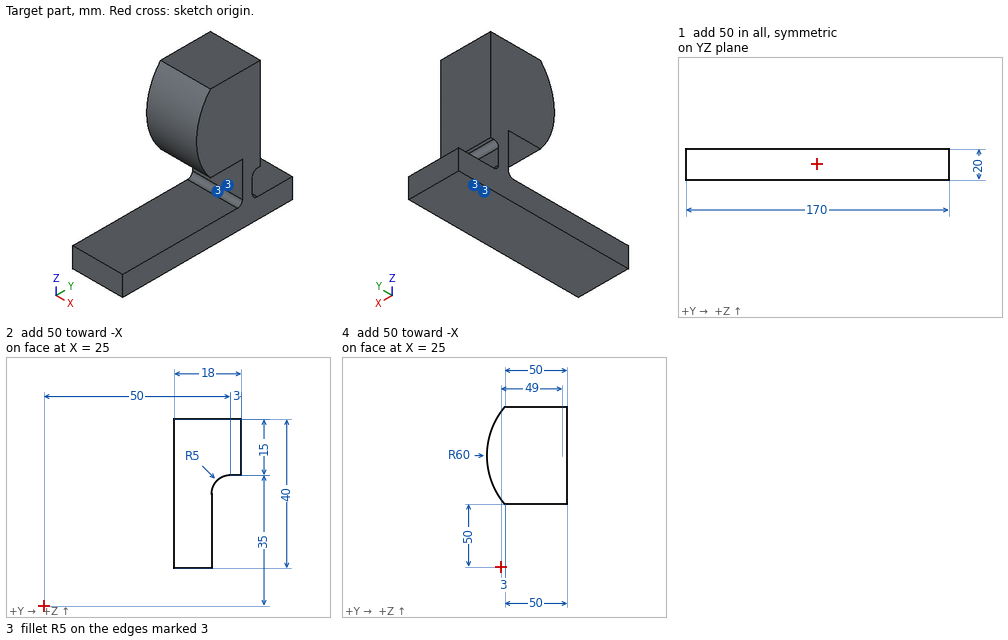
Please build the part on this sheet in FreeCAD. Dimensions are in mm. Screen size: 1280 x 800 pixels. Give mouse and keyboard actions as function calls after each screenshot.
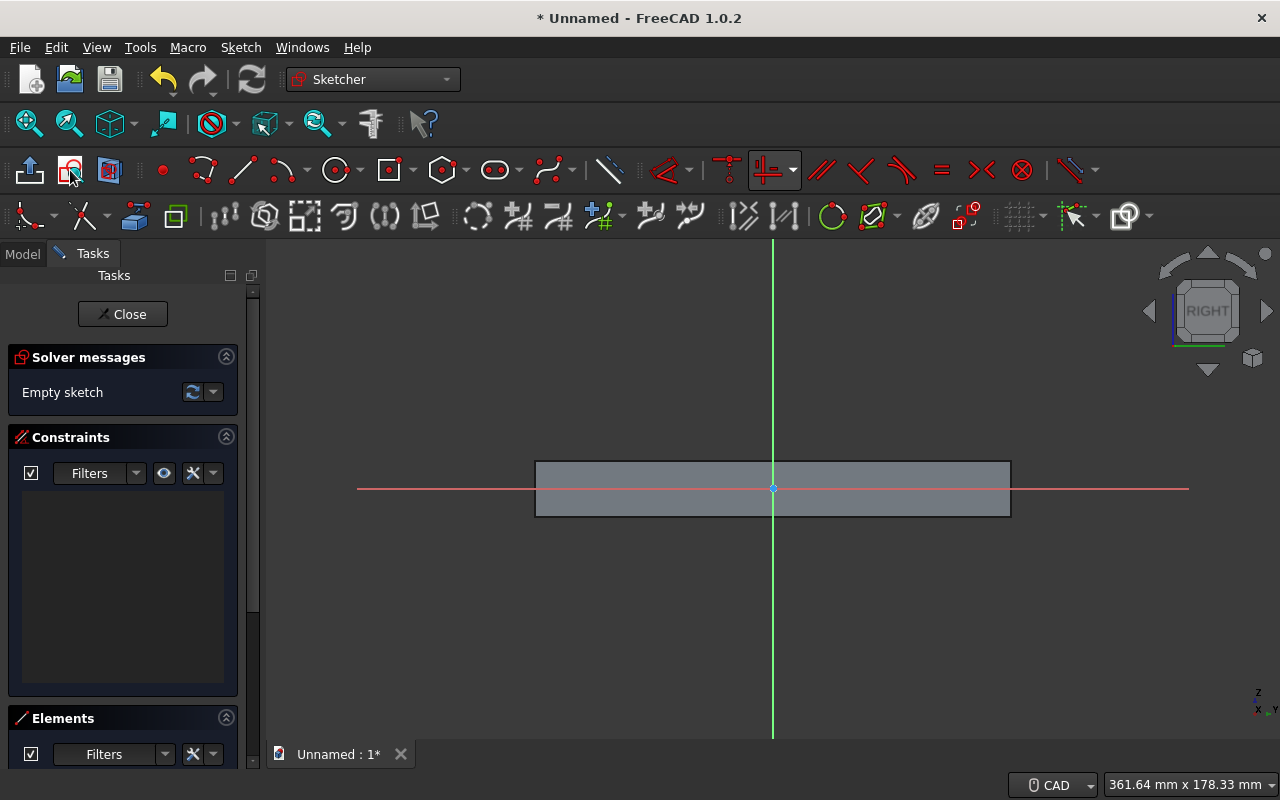
scroll(964, 362, up, 4)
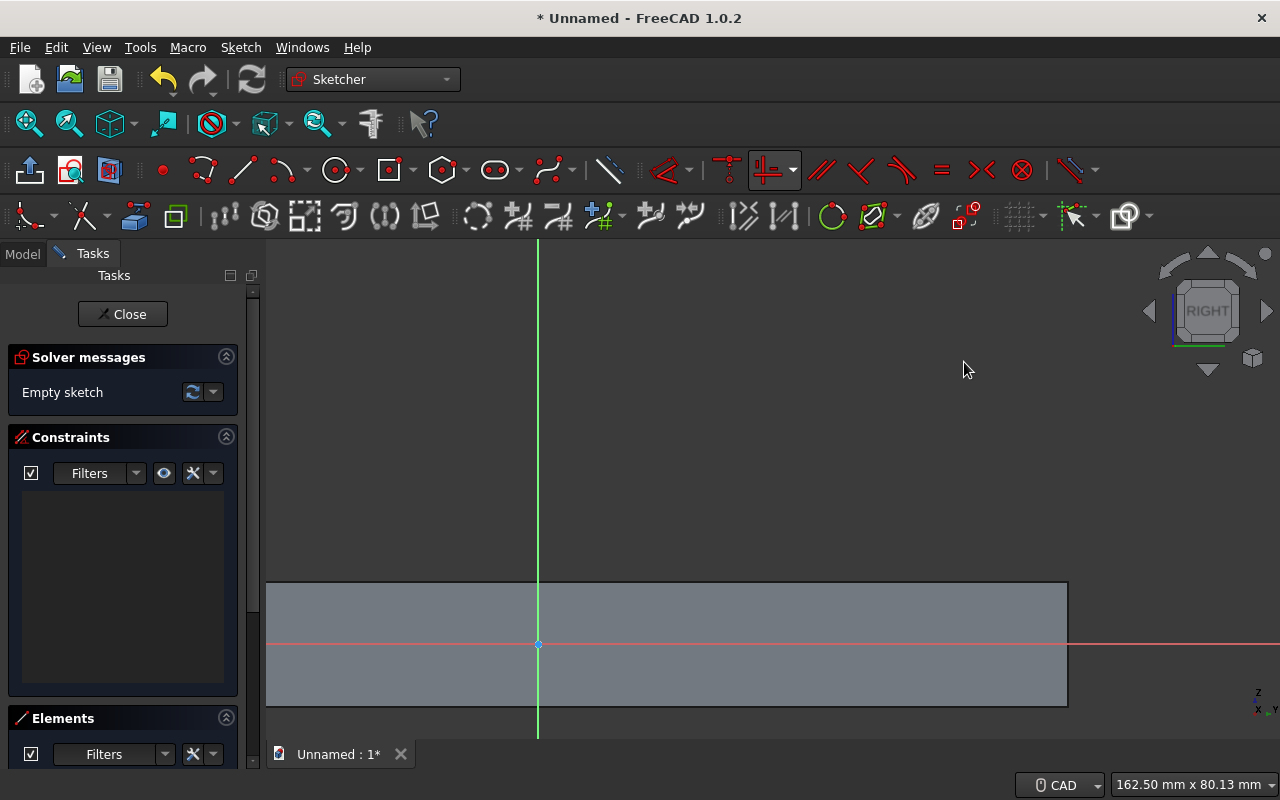
click(204, 170)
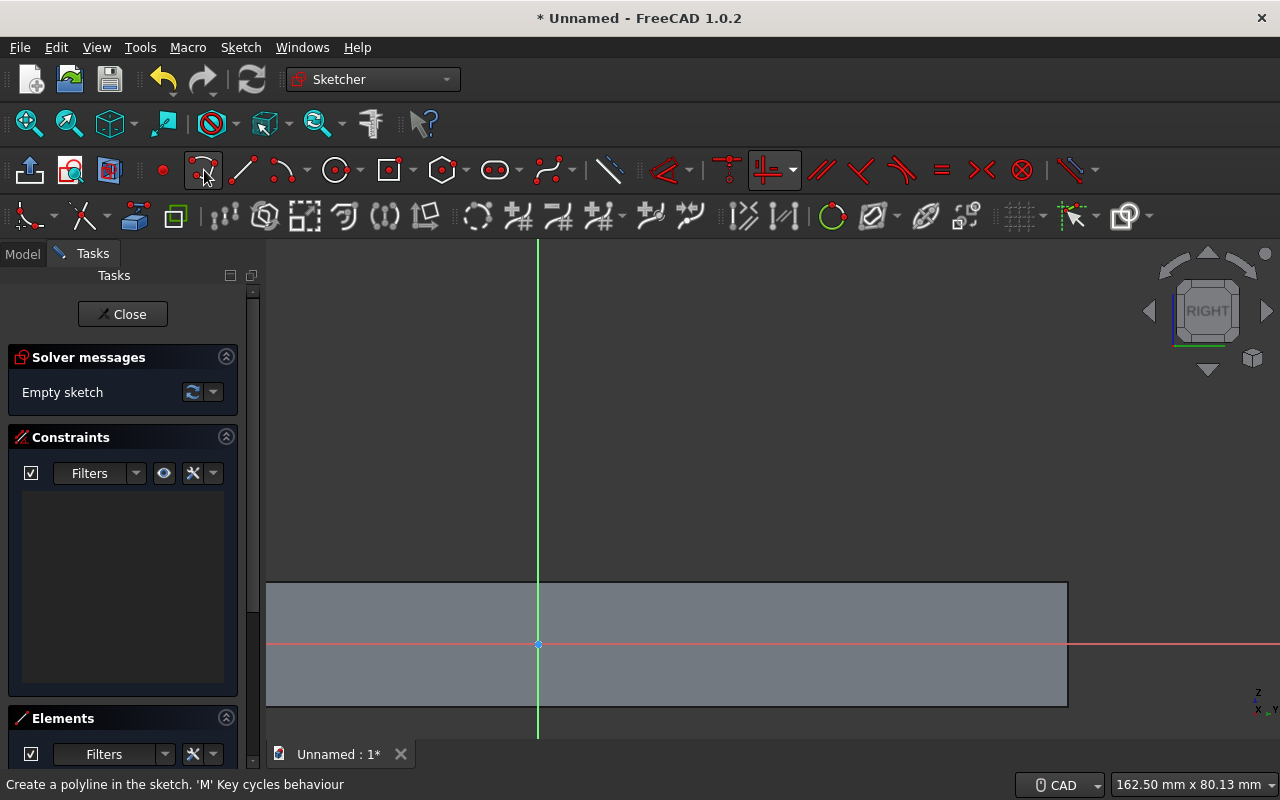
click(850, 426)
click(869, 426)
click(869, 332)
click(756, 332)
click(756, 582)
click(819, 582)
click(819, 457)
right_click(819, 457)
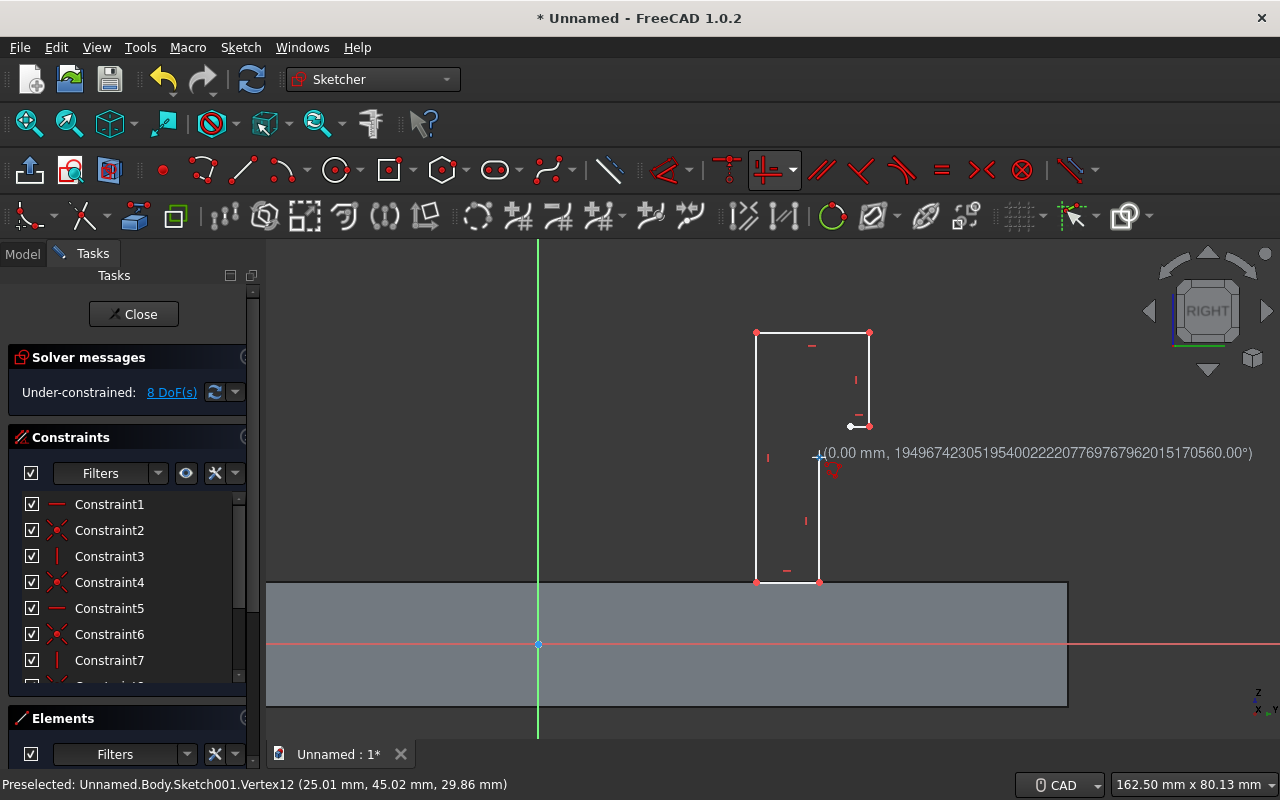
key(g)
key(3)
key(a)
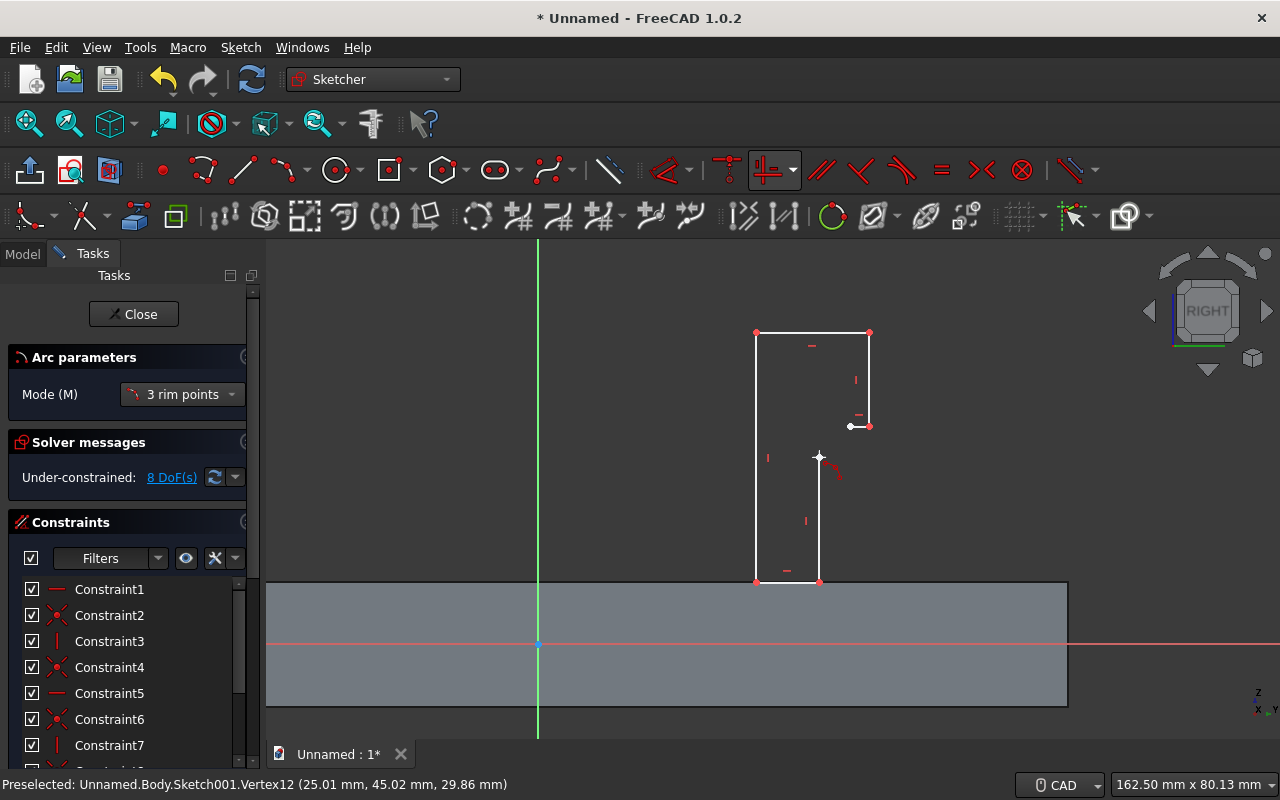
click(819, 458)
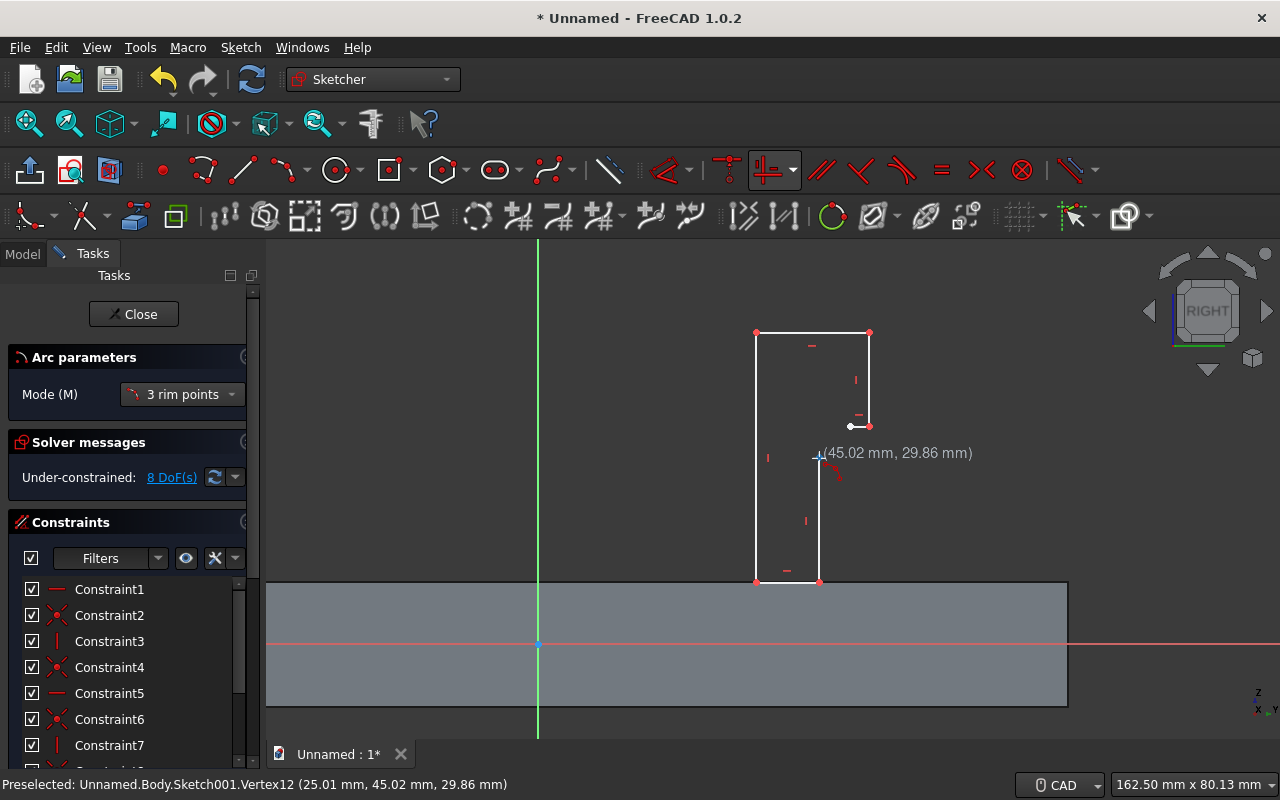
scroll(850, 426, up, 3)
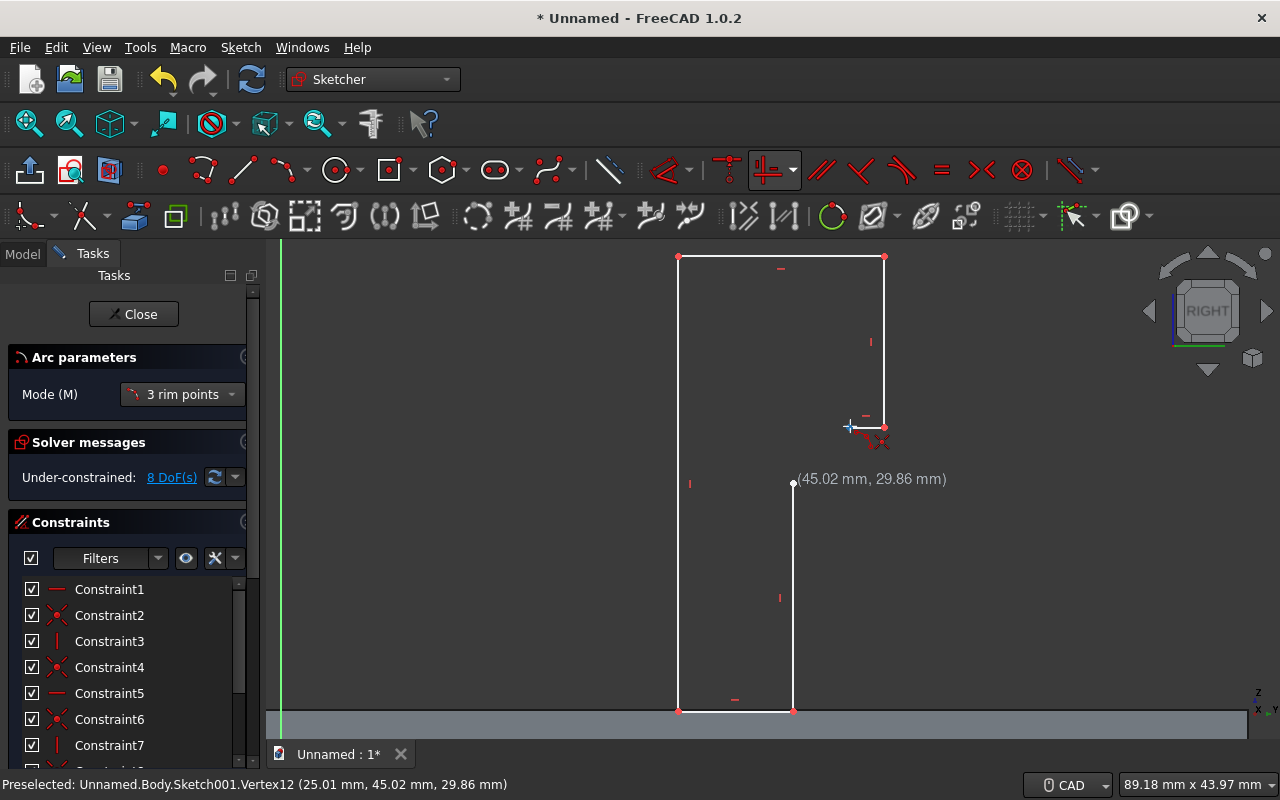
click(850, 428)
click(809, 442)
key(Escape)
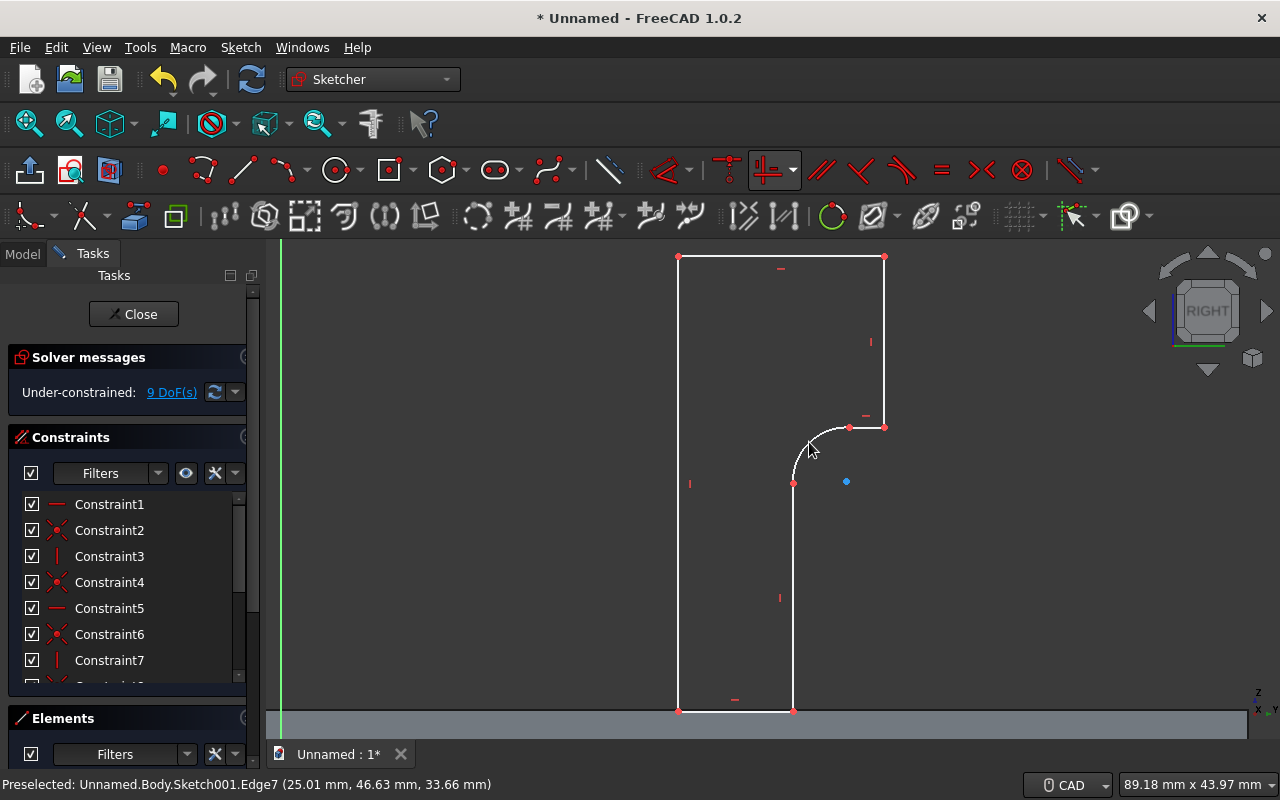
scroll(860, 428, up, 2)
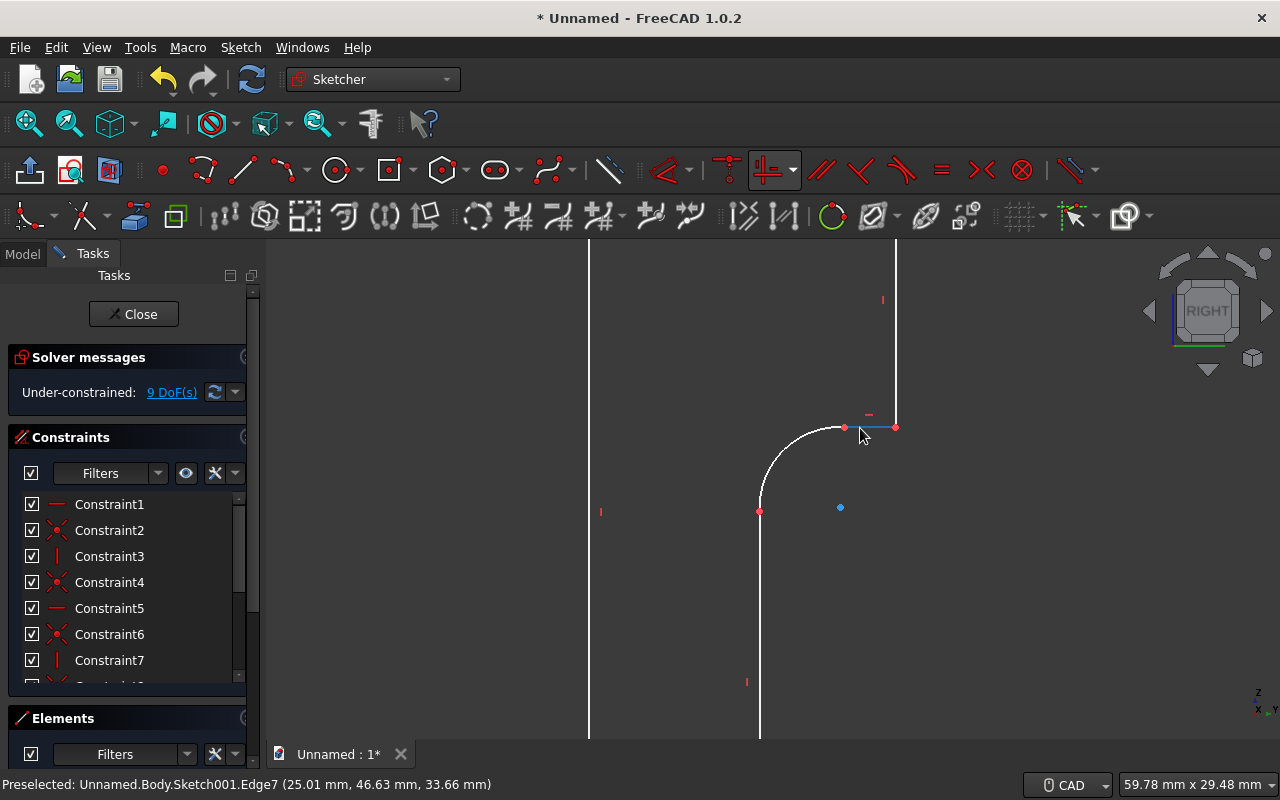
click(860, 427)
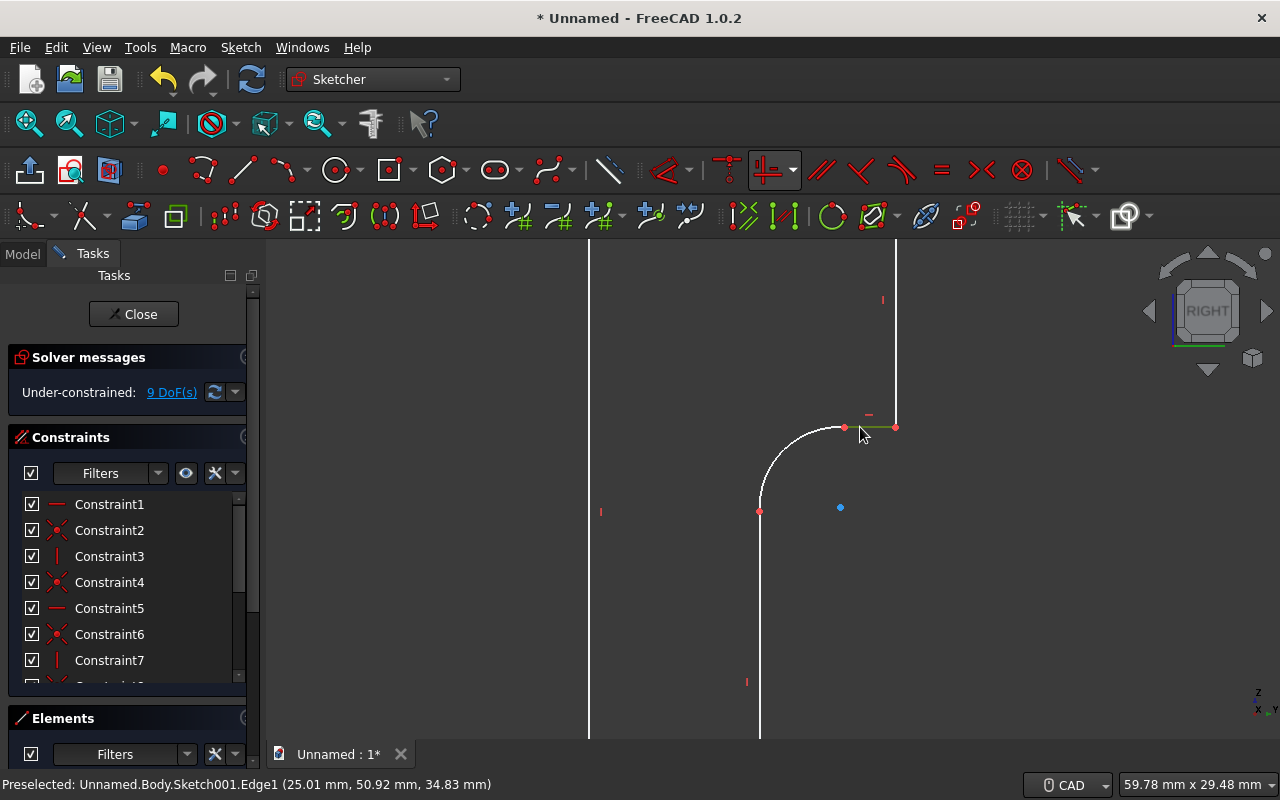
click(805, 435)